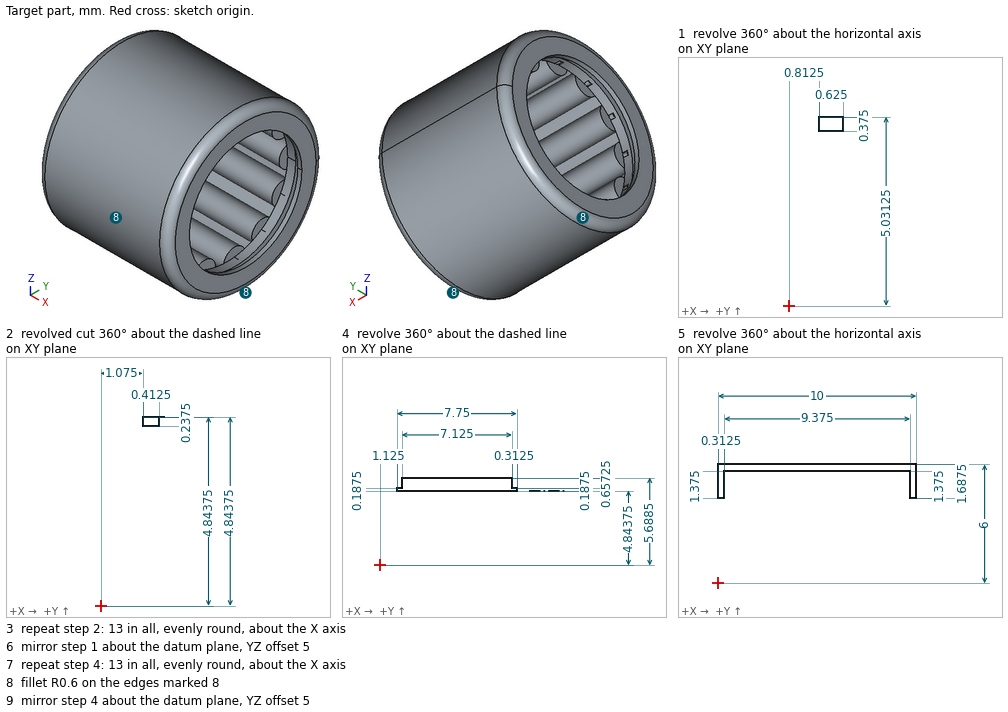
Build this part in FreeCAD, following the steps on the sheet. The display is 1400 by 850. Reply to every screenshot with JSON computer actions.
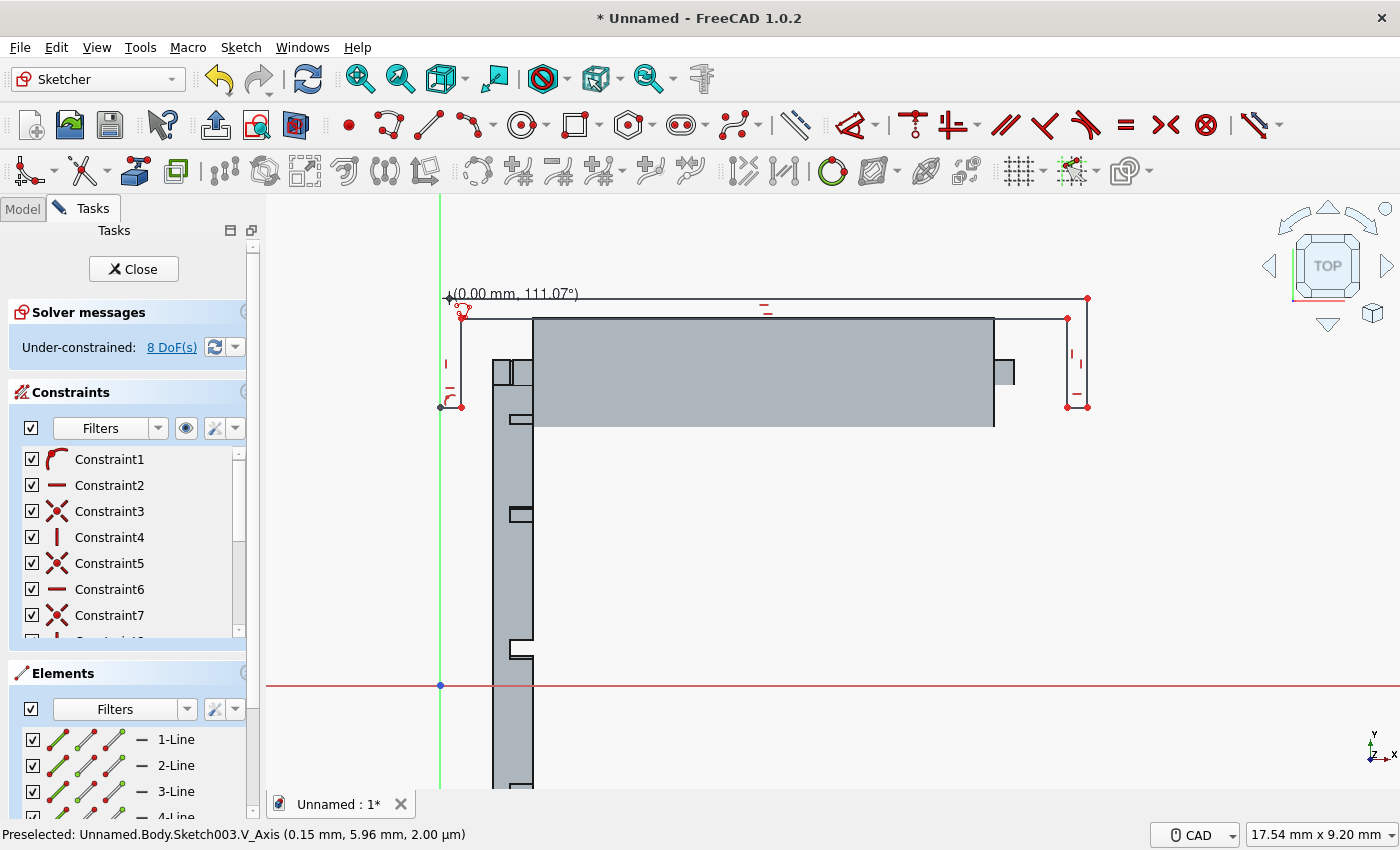
{"action": "scroll", "coordinate": [440, 407], "scroll_direction": "up", "scroll_amount": 3}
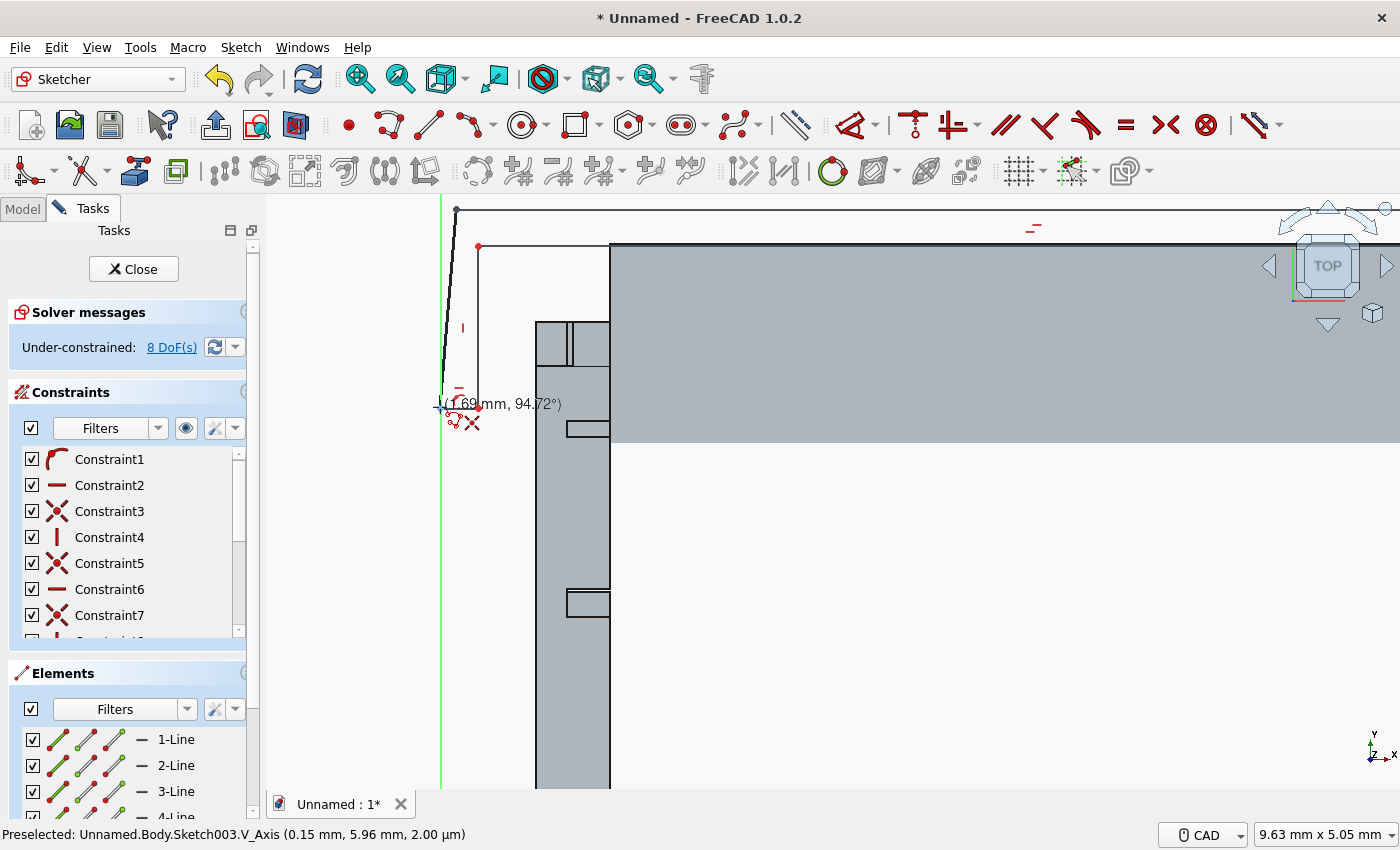
{"action": "left_click", "coordinate": [441, 409]}
{"action": "key", "text": "Escape"}
{"action": "key", "text": "Escape"}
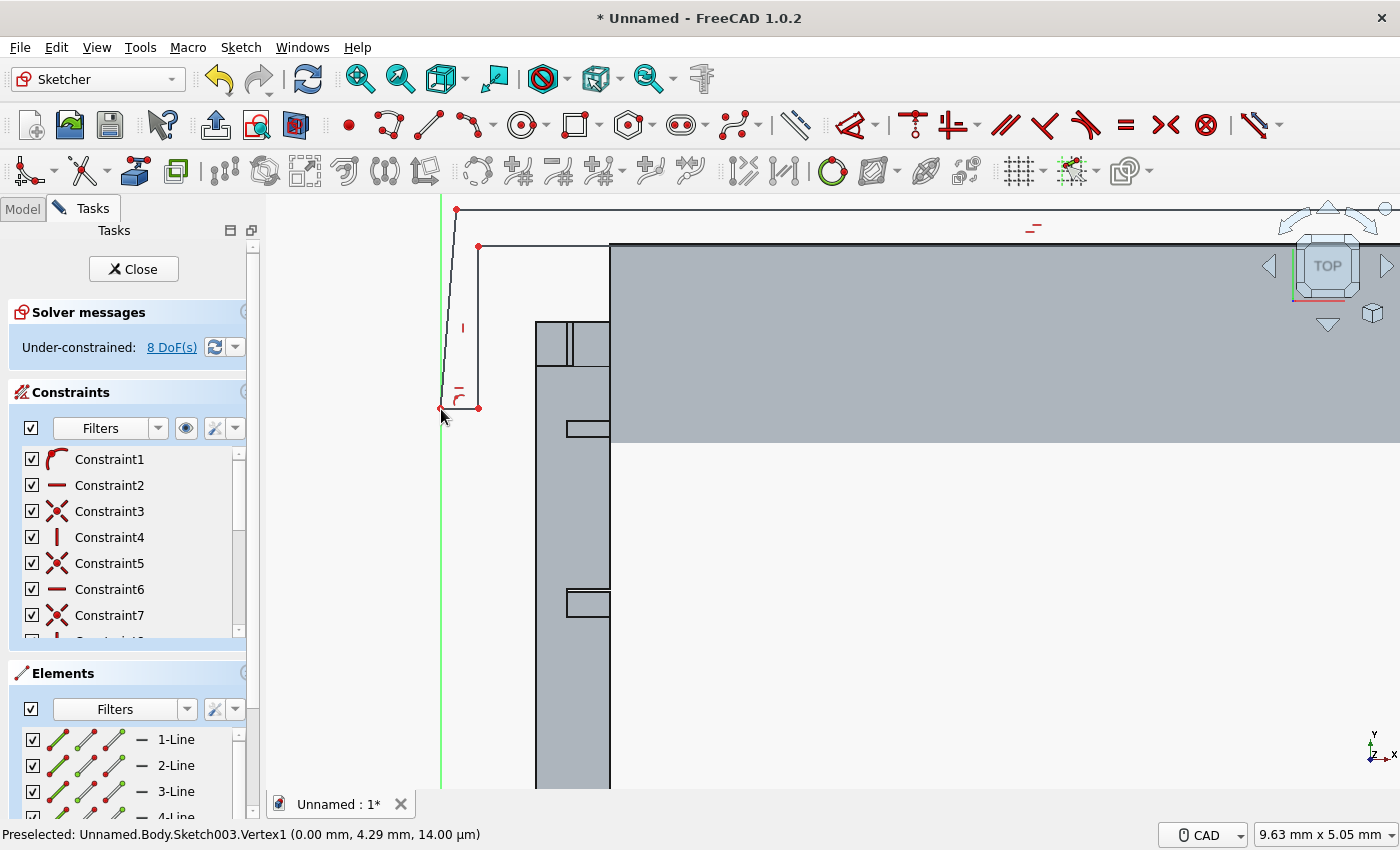
{"action": "scroll", "coordinate": [452, 269], "scroll_direction": "up", "scroll_amount": 2}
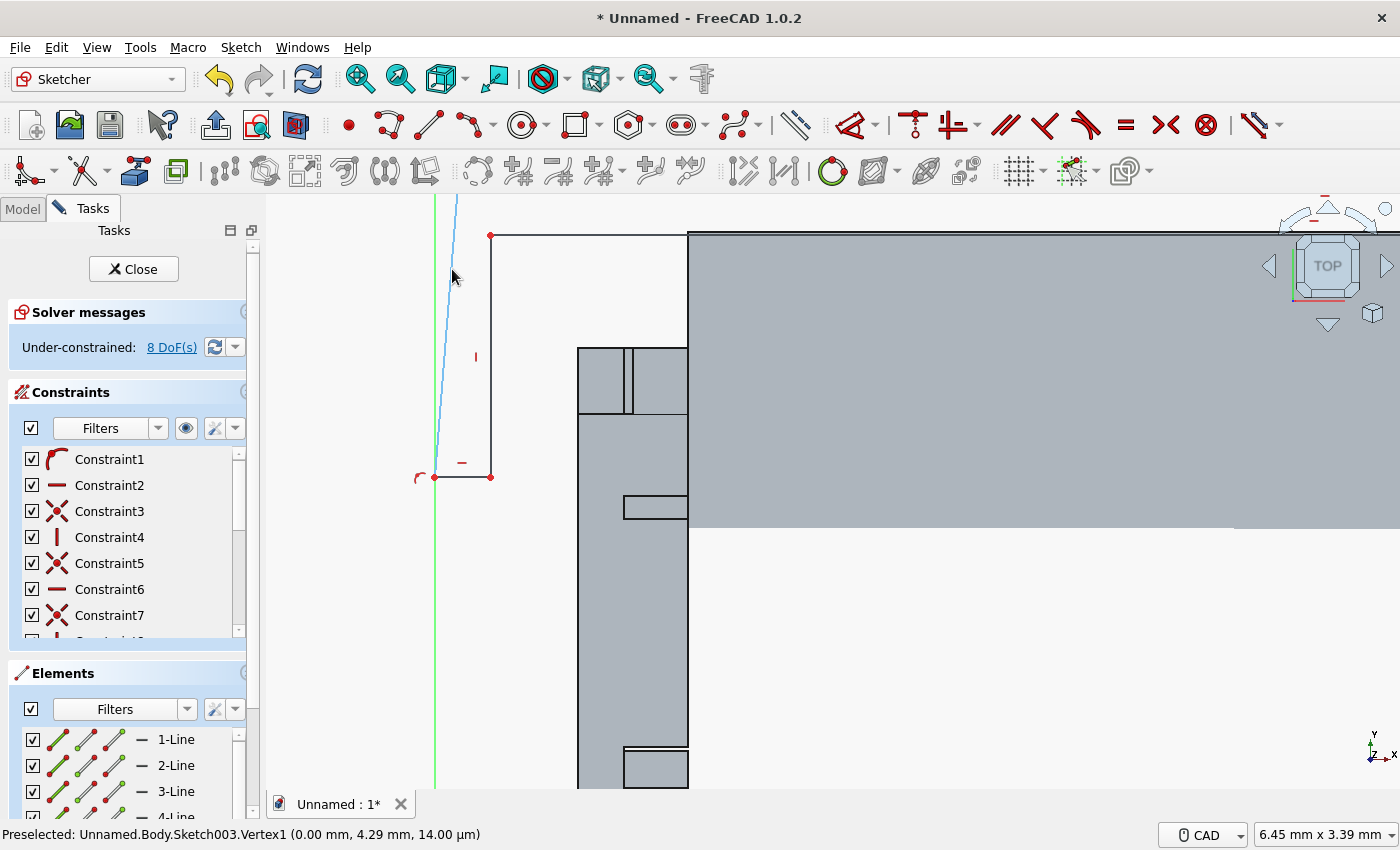
{"action": "left_click", "coordinate": [451, 270]}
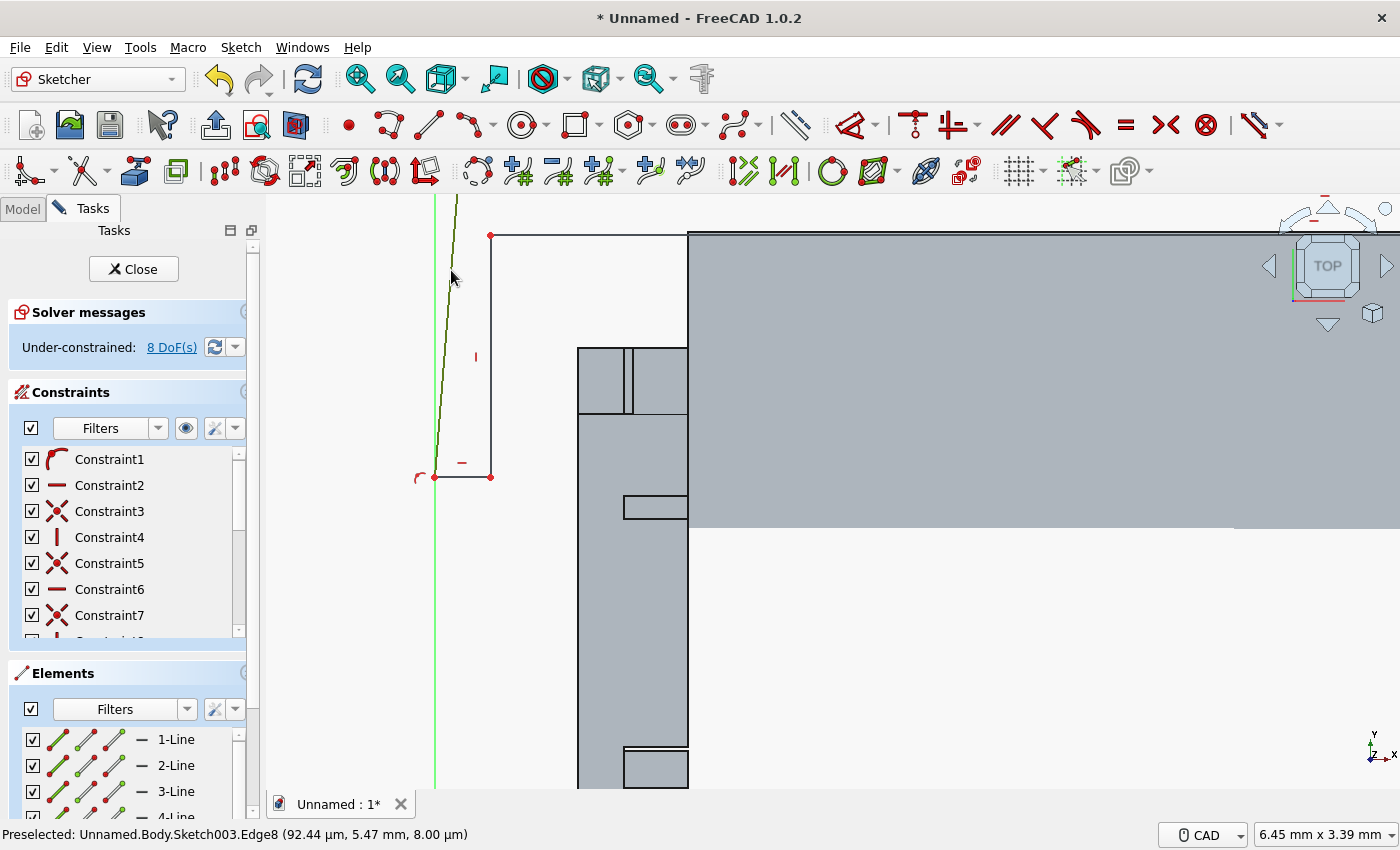
{"action": "left_click", "coordinate": [980, 126]}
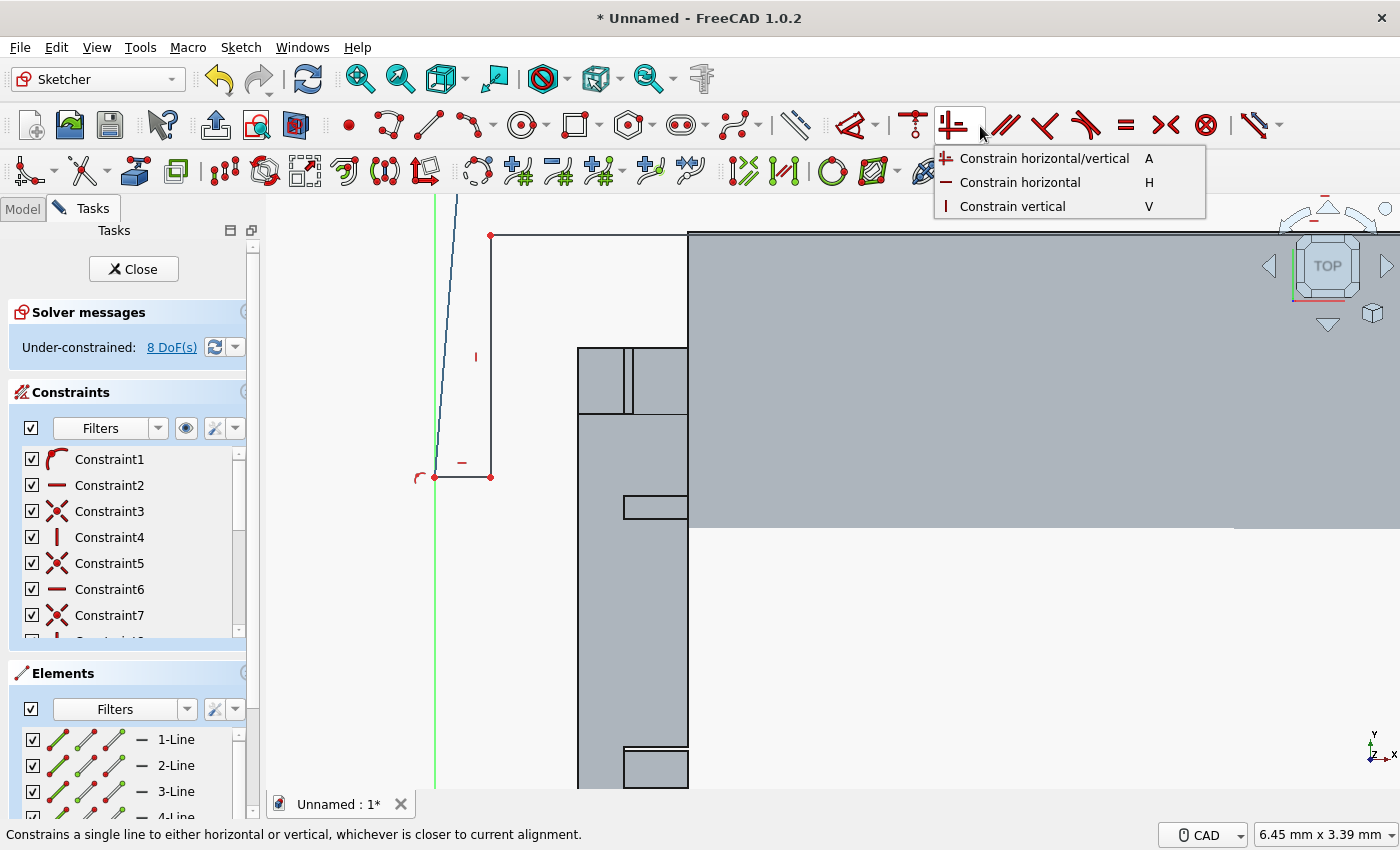
{"action": "left_click", "coordinate": [1070, 206]}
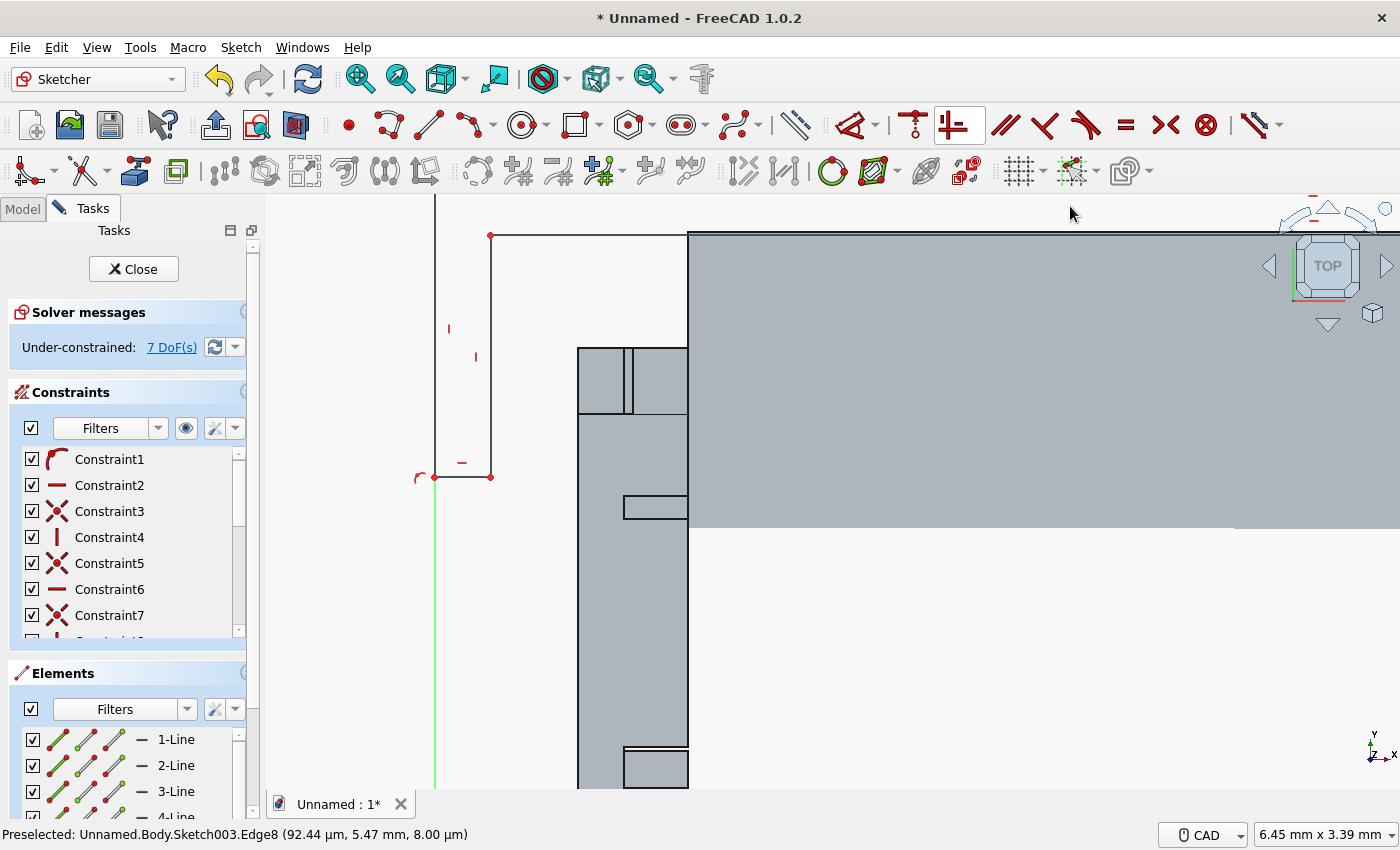
{"action": "left_click", "coordinate": [850, 126]}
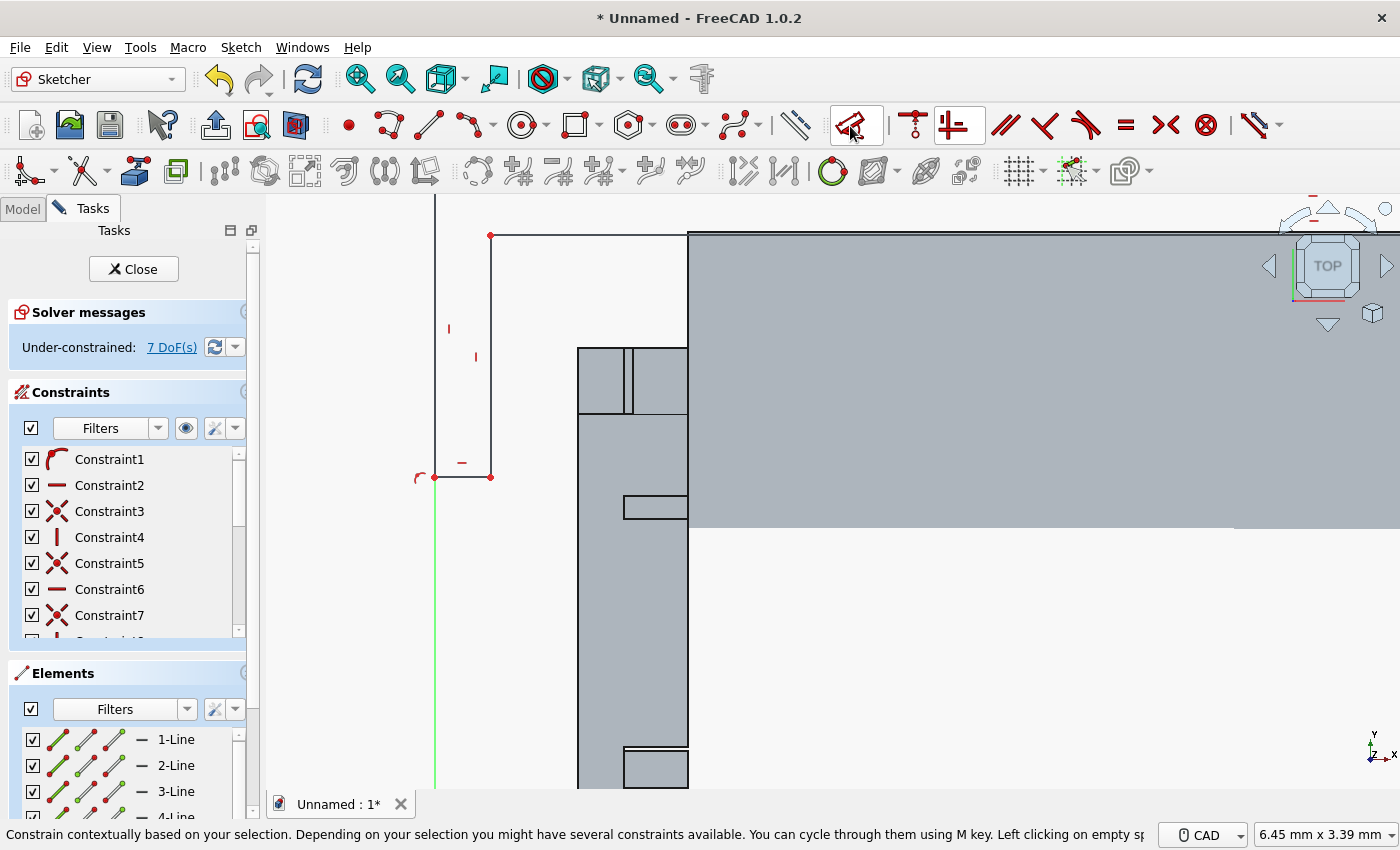
{"action": "scroll", "coordinate": [445, 367], "scroll_direction": "down", "scroll_amount": 5}